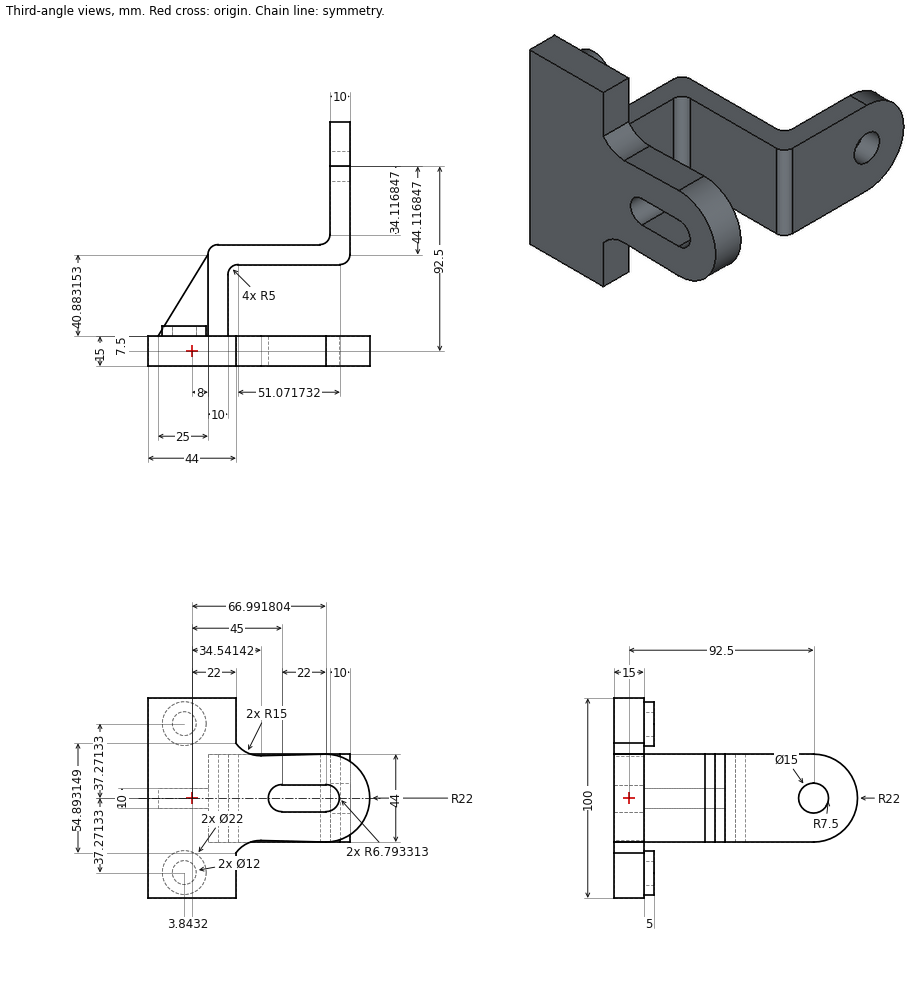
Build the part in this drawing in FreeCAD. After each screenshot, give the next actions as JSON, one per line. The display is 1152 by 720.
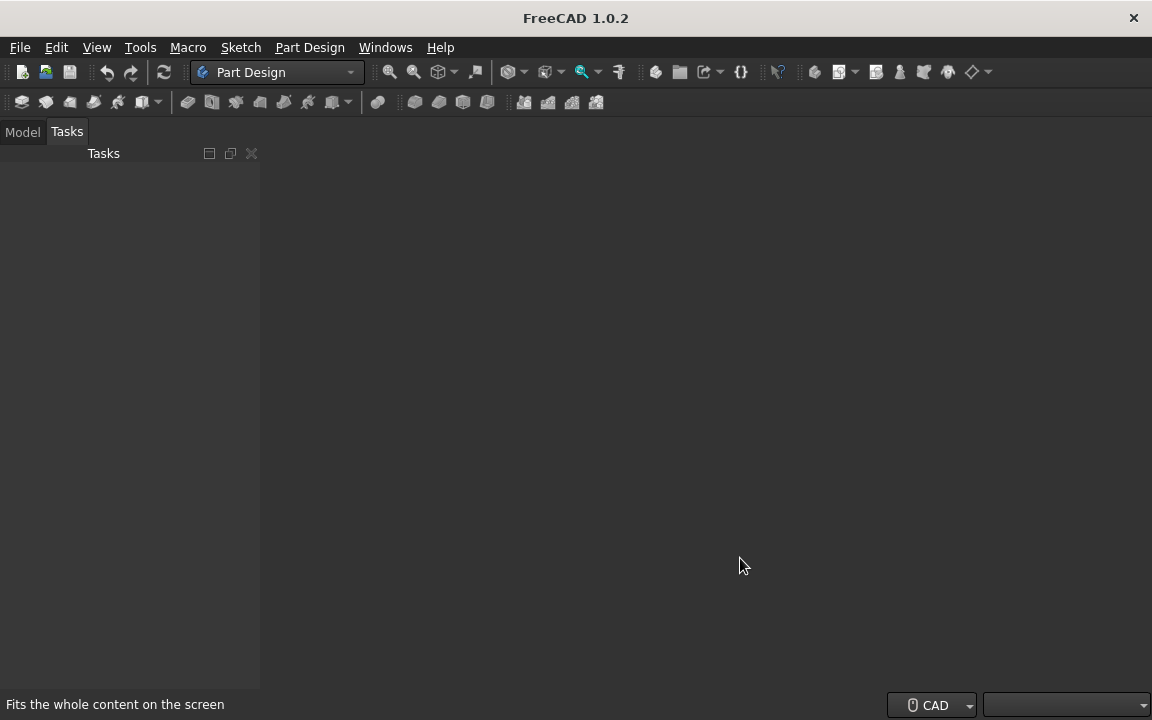
{"action": "left_click", "coordinate": [22, 72]}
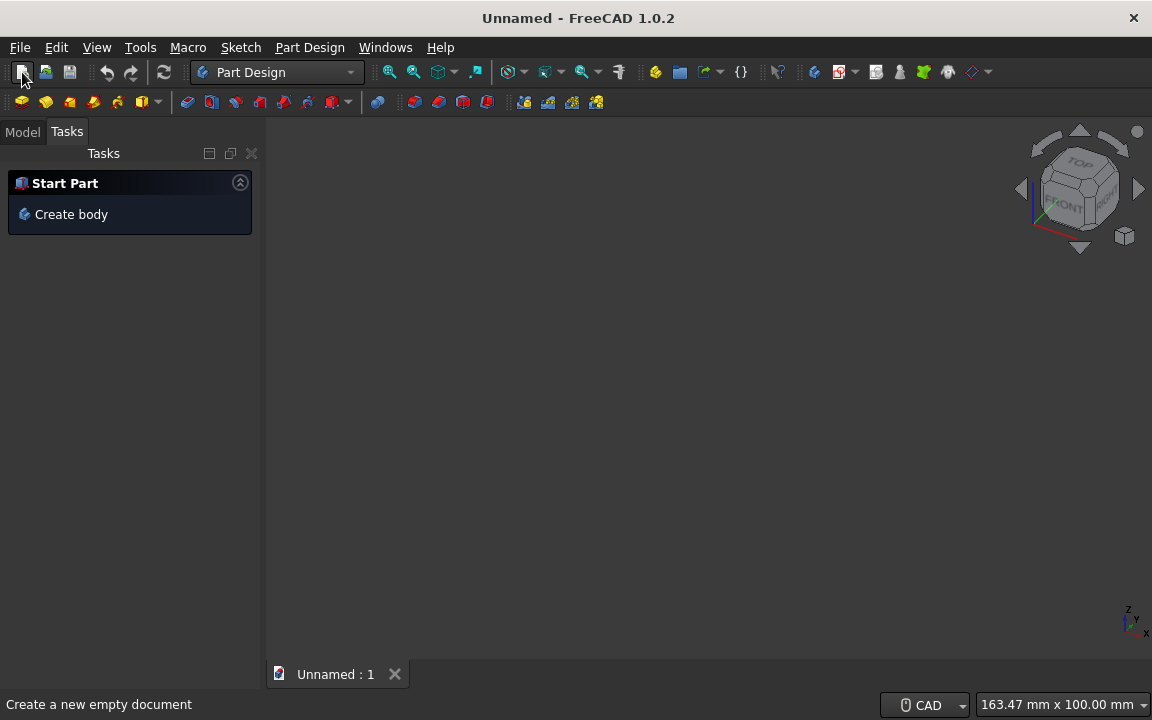
{"action": "left_click", "coordinate": [840, 72]}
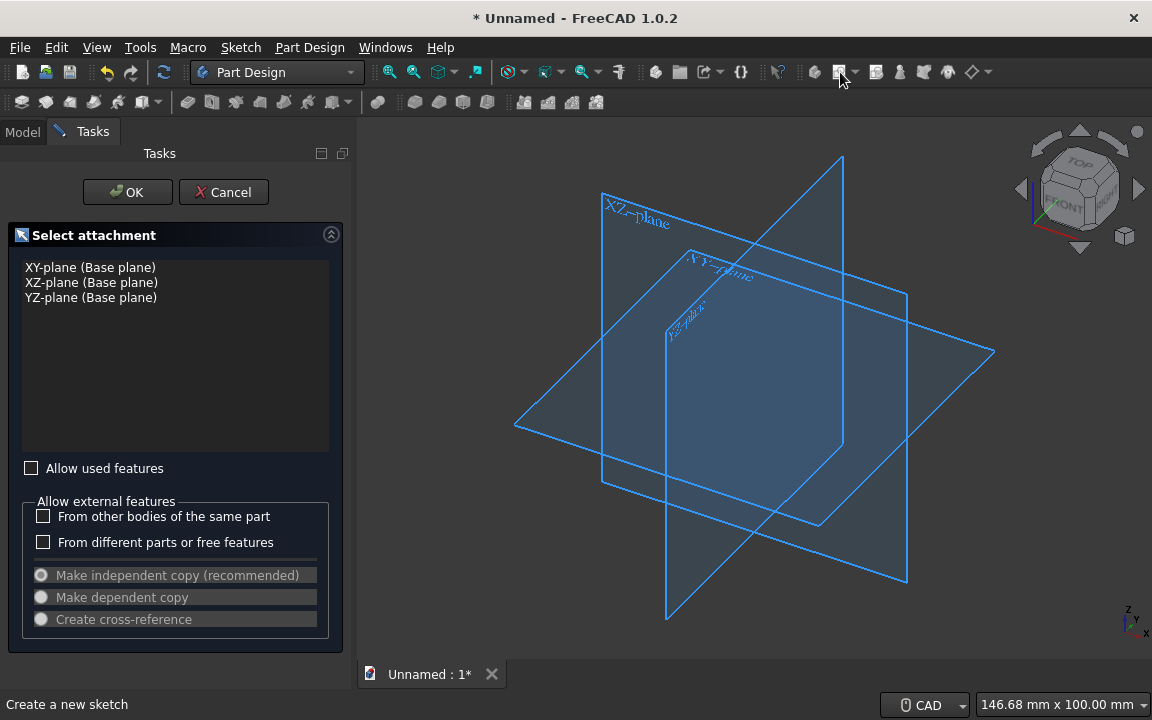
{"action": "left_click", "coordinate": [82, 268]}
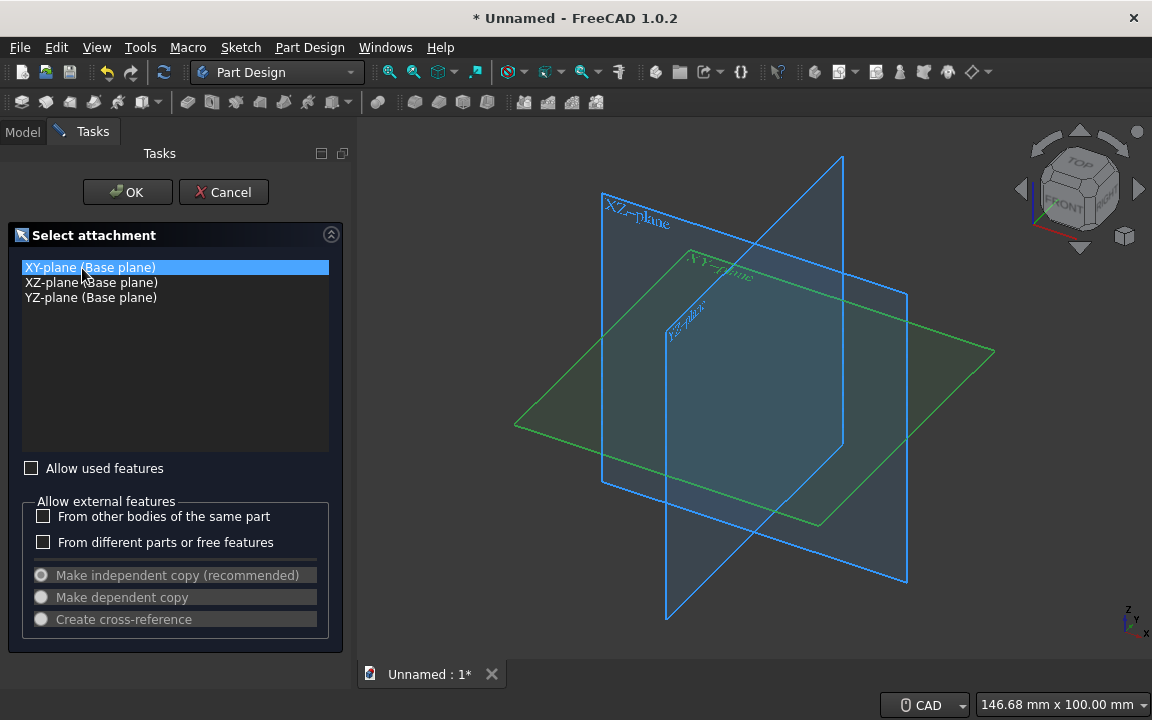
{"action": "left_click", "coordinate": [128, 192]}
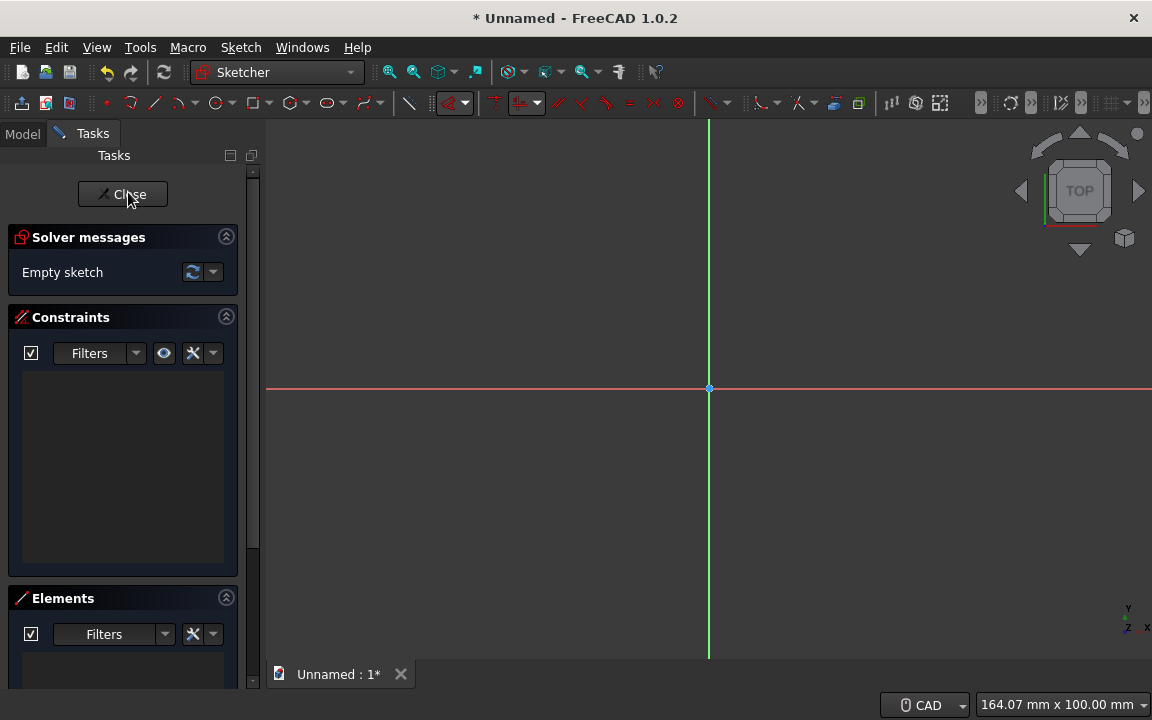
{"action": "scroll", "coordinate": [765, 389], "scroll_direction": "up", "scroll_amount": 4}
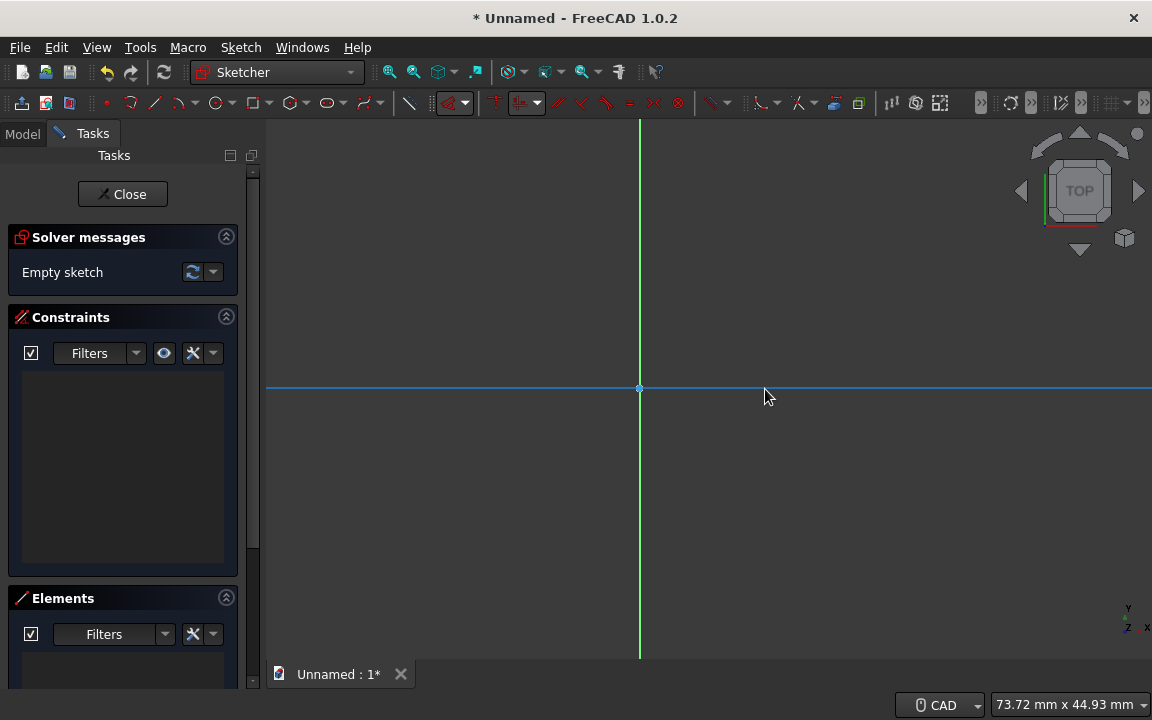
{"action": "left_click", "coordinate": [272, 104]}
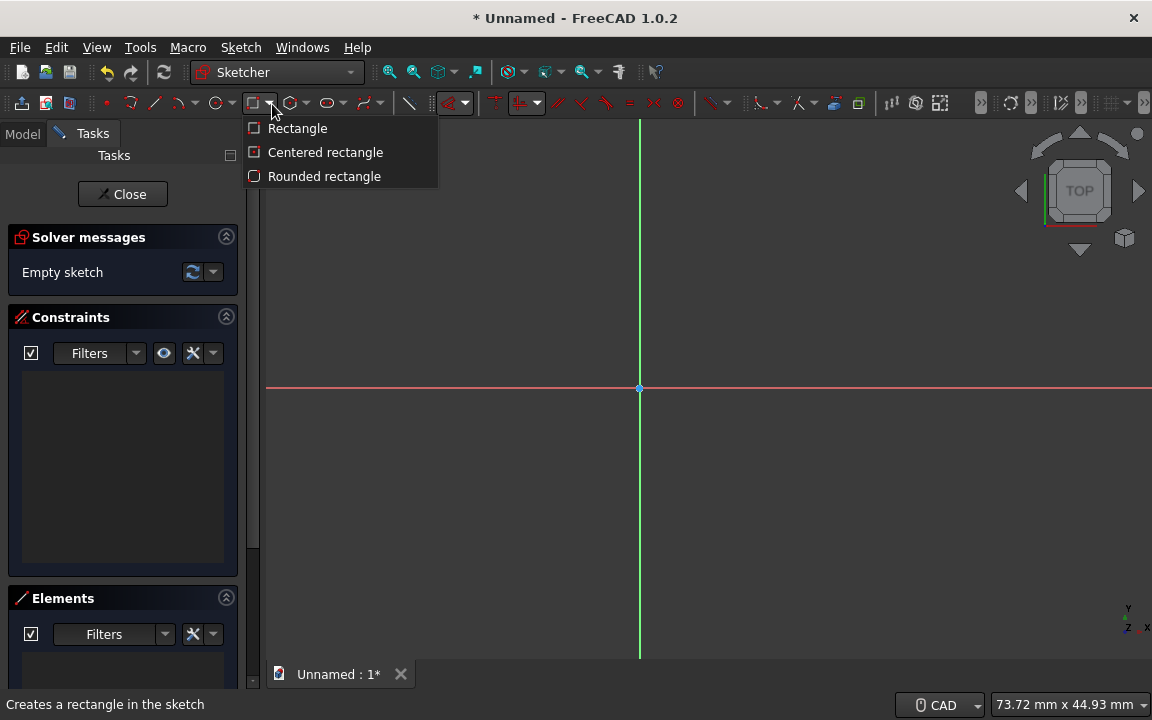
{"action": "left_click", "coordinate": [340, 152]}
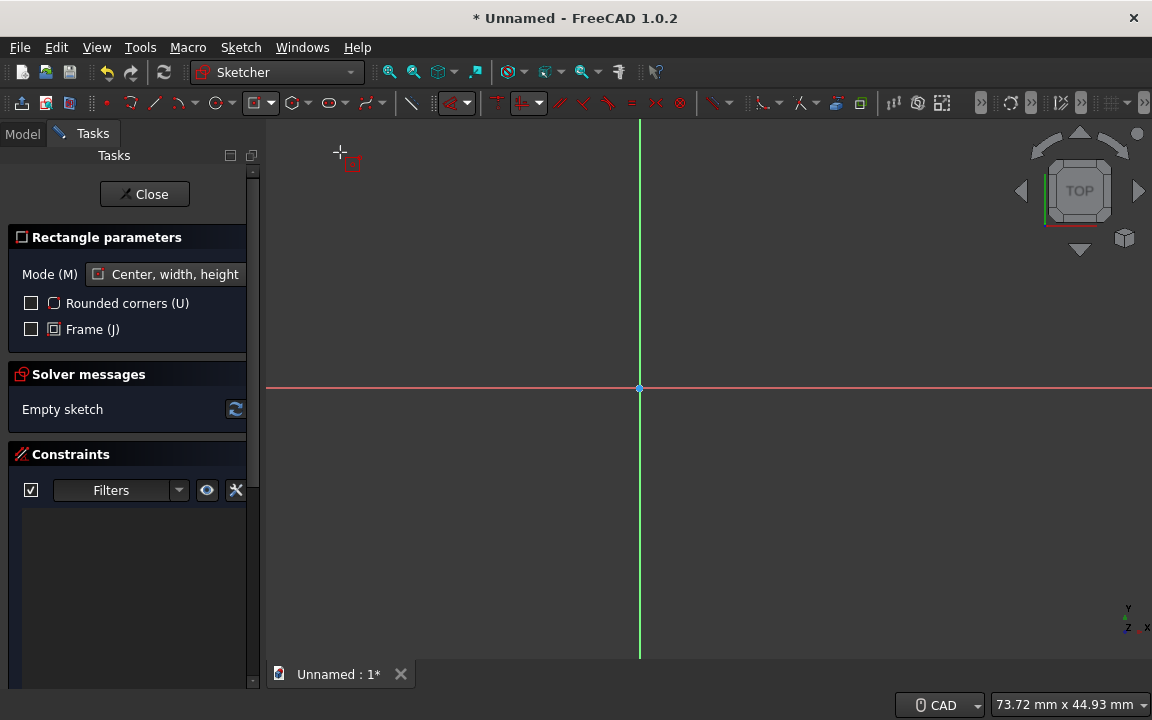
{"action": "left_click", "coordinate": [640, 388]}
{"action": "mouse_move", "coordinate": [904, 298]}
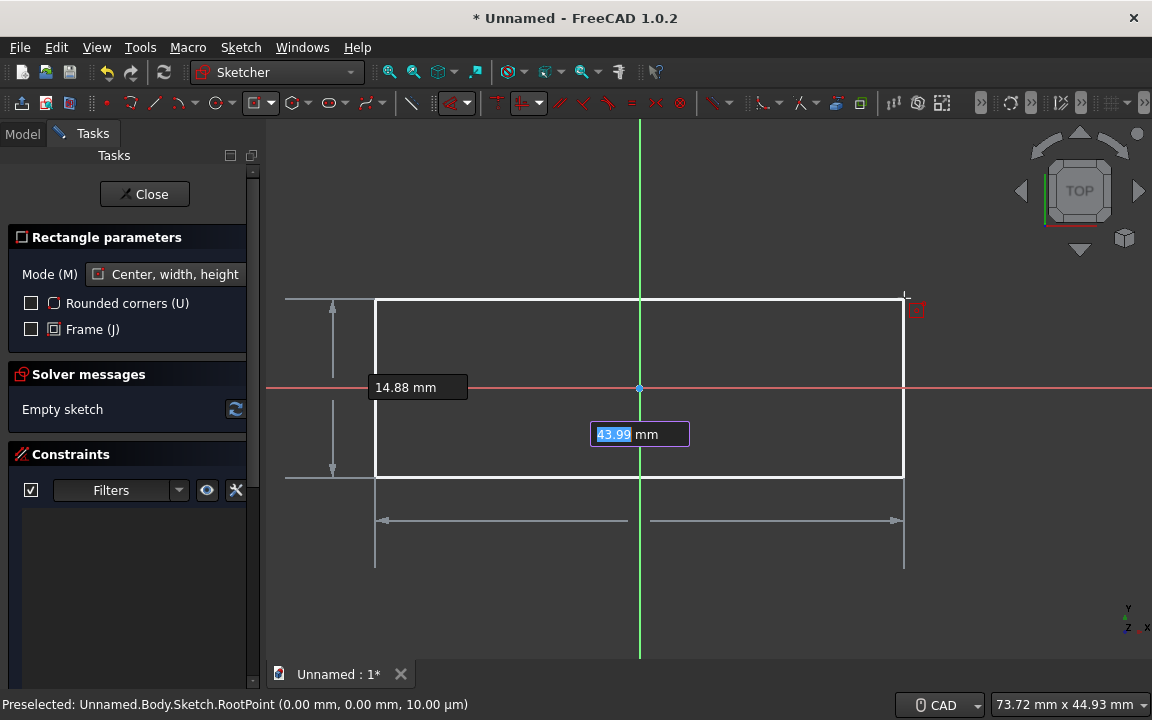
{"action": "type", "text": "44"}
{"action": "key", "text": "Tab"}
{"action": "type", "text": "15"}
{"action": "key", "text": "Return"}
{"action": "key", "text": "Escape"}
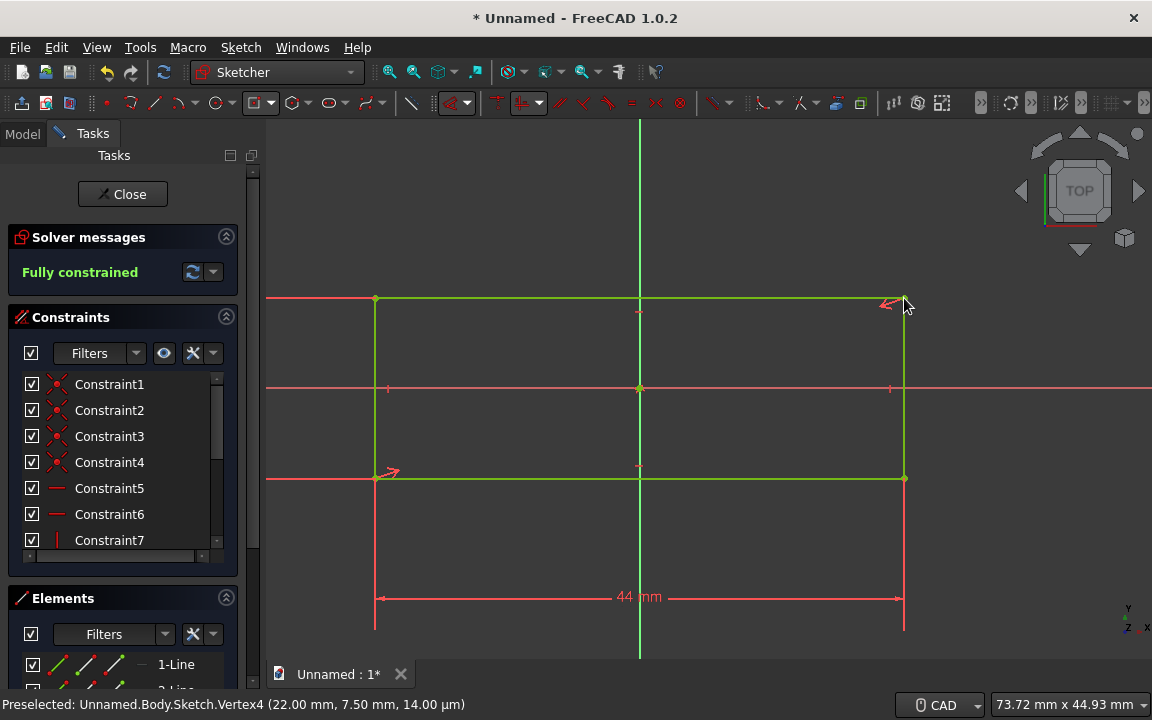
{"action": "left_click", "coordinate": [123, 194]}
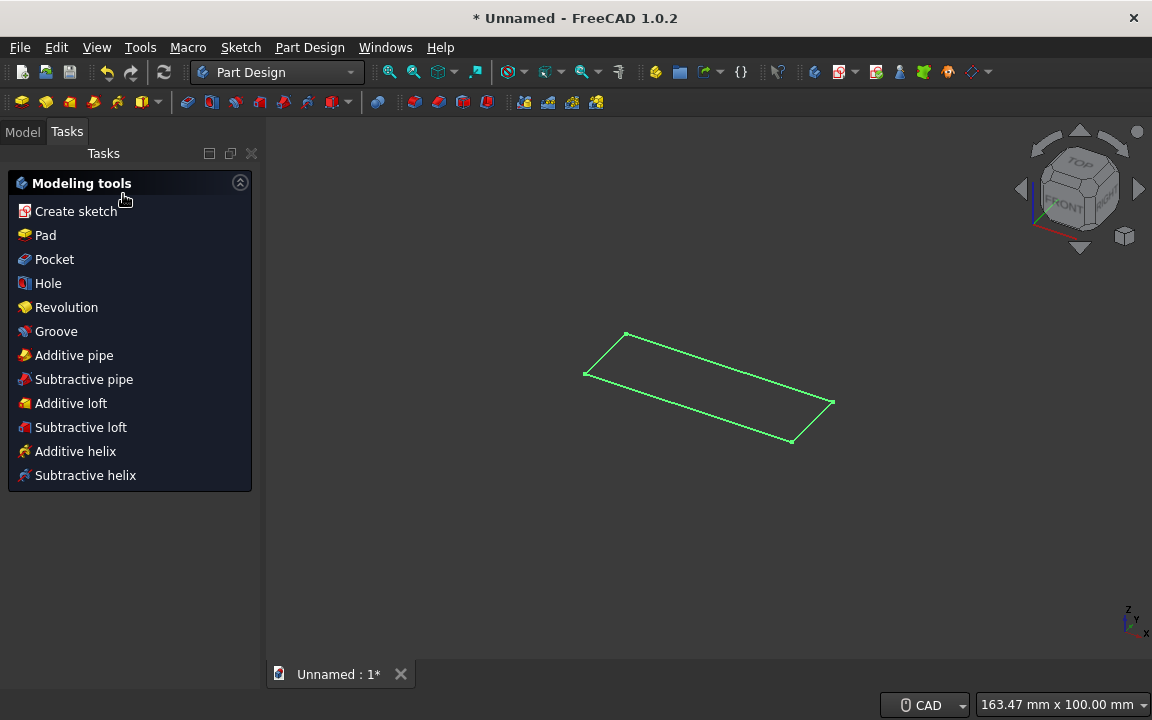
{"action": "left_click", "coordinate": [22, 102]}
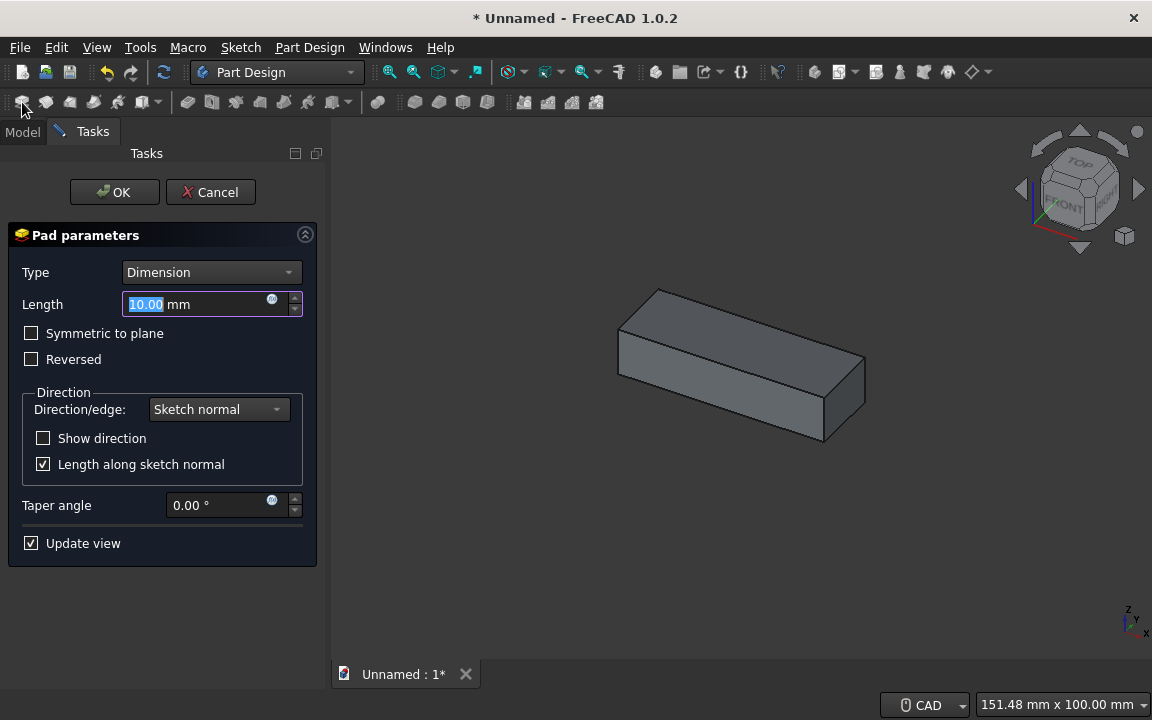
{"action": "type", "text": "100"}
{"action": "key", "text": "Tab"}